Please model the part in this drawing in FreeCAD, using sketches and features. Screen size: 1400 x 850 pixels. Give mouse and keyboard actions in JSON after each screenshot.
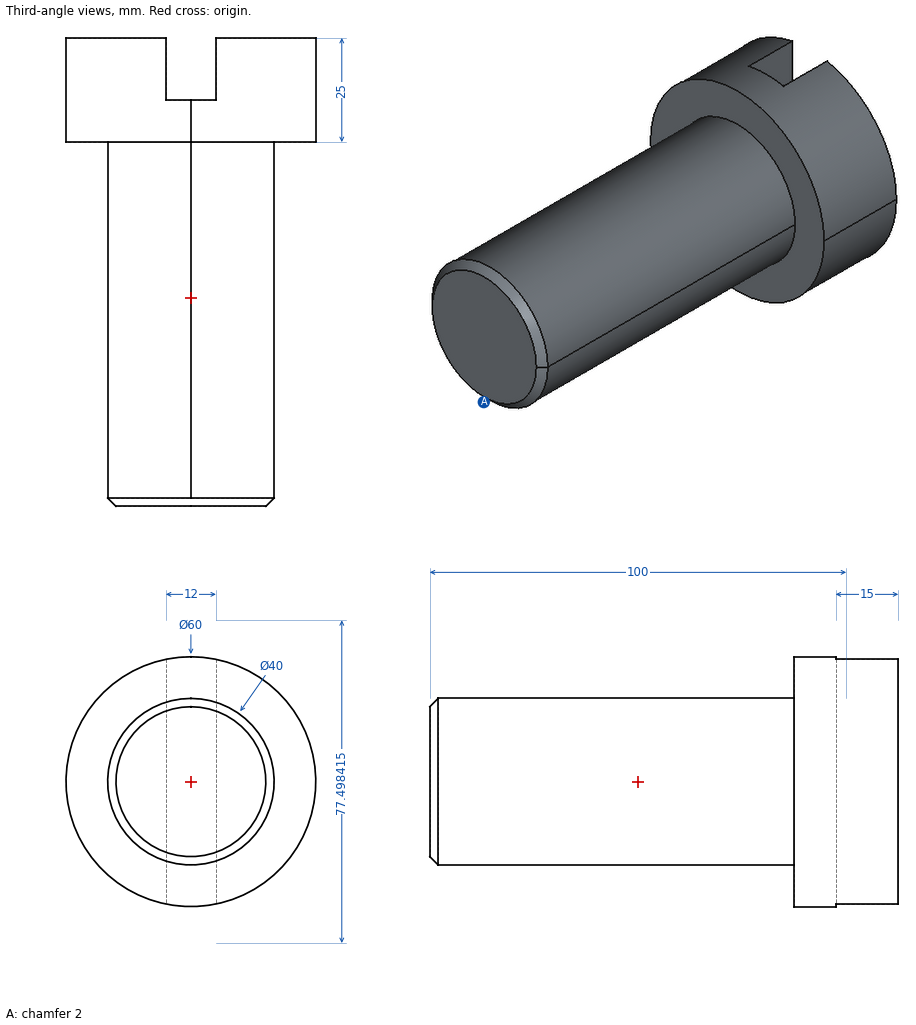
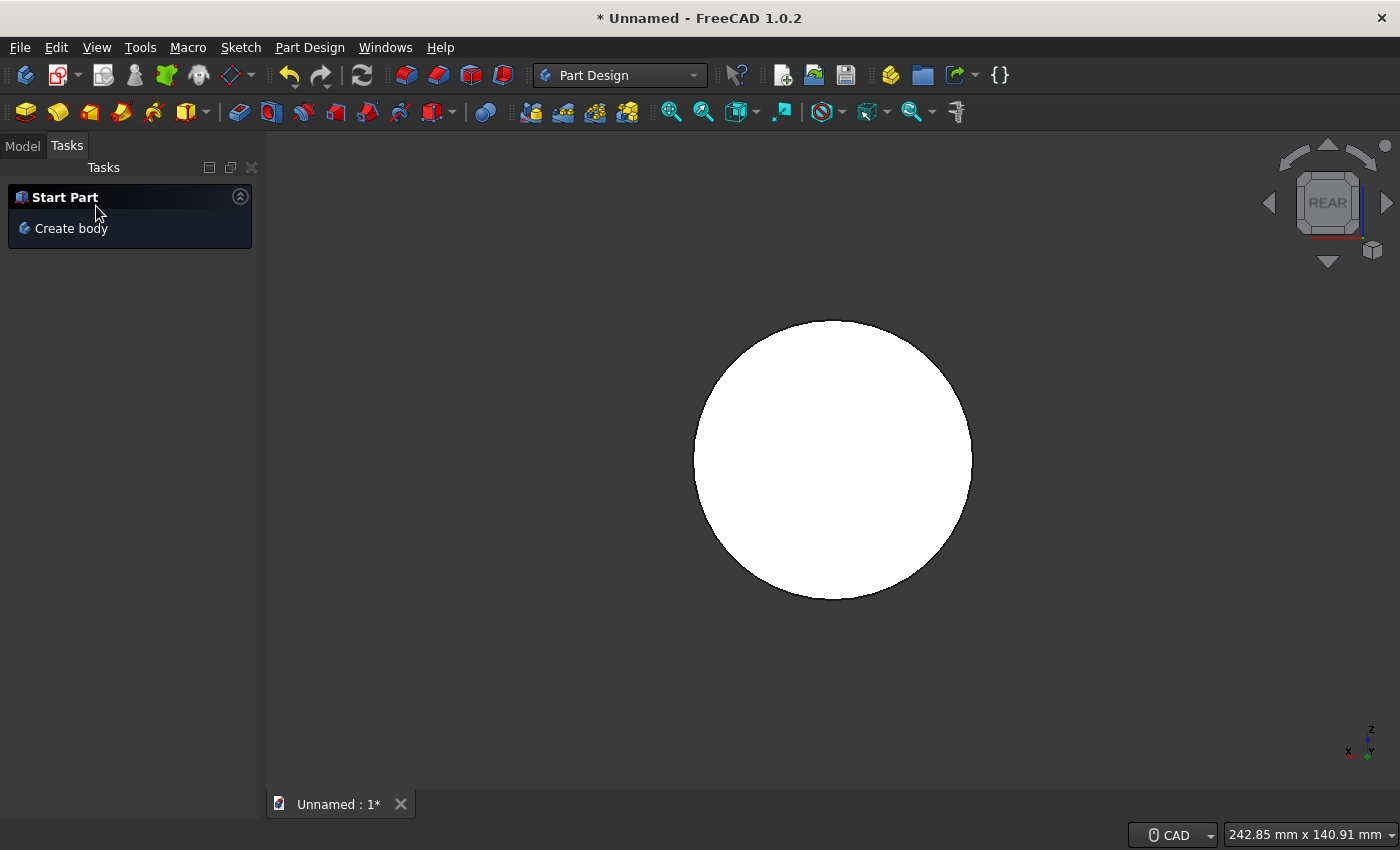
{"action": "left_click", "coordinate": [672, 112]}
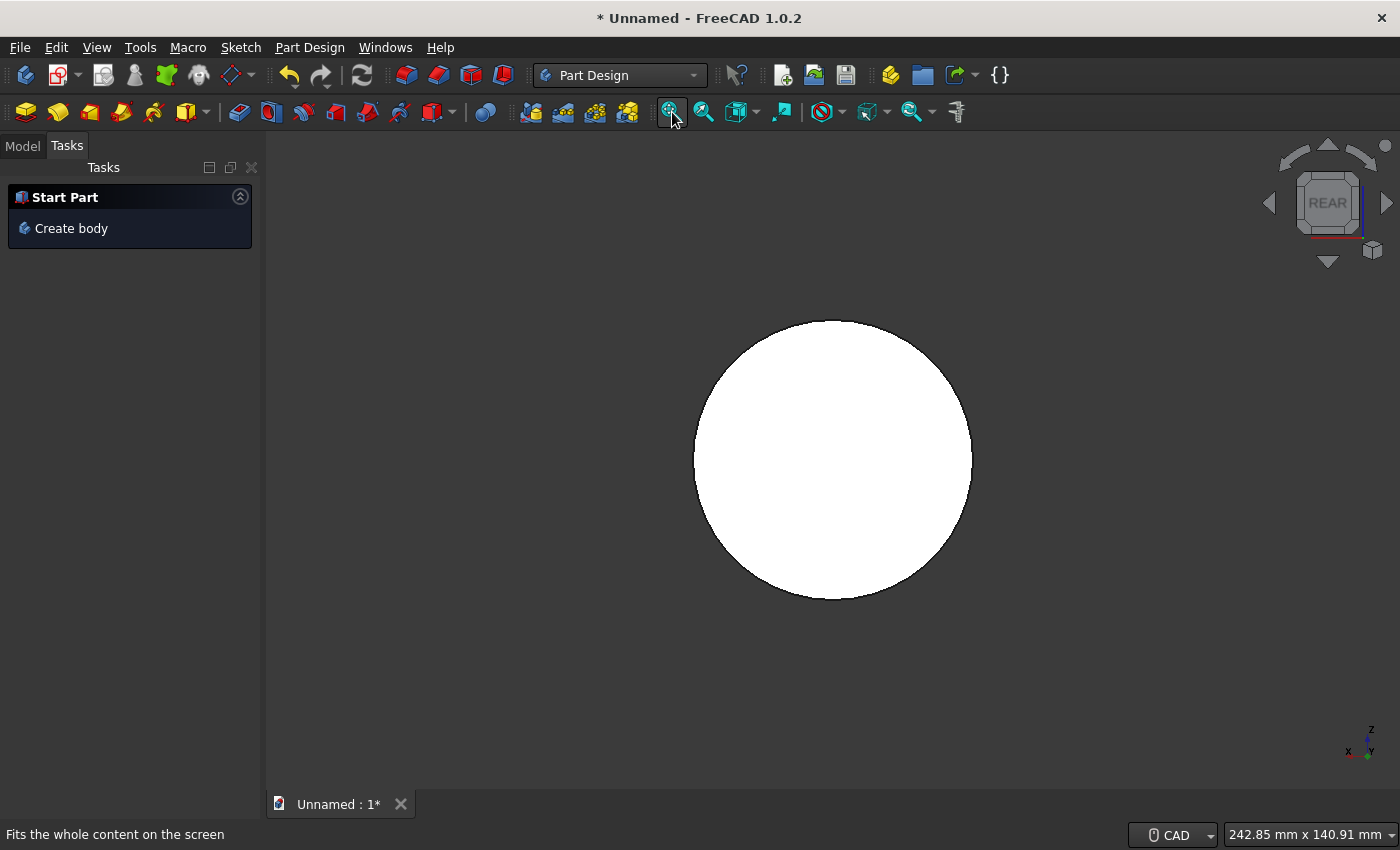
{"action": "left_click", "coordinate": [833, 459]}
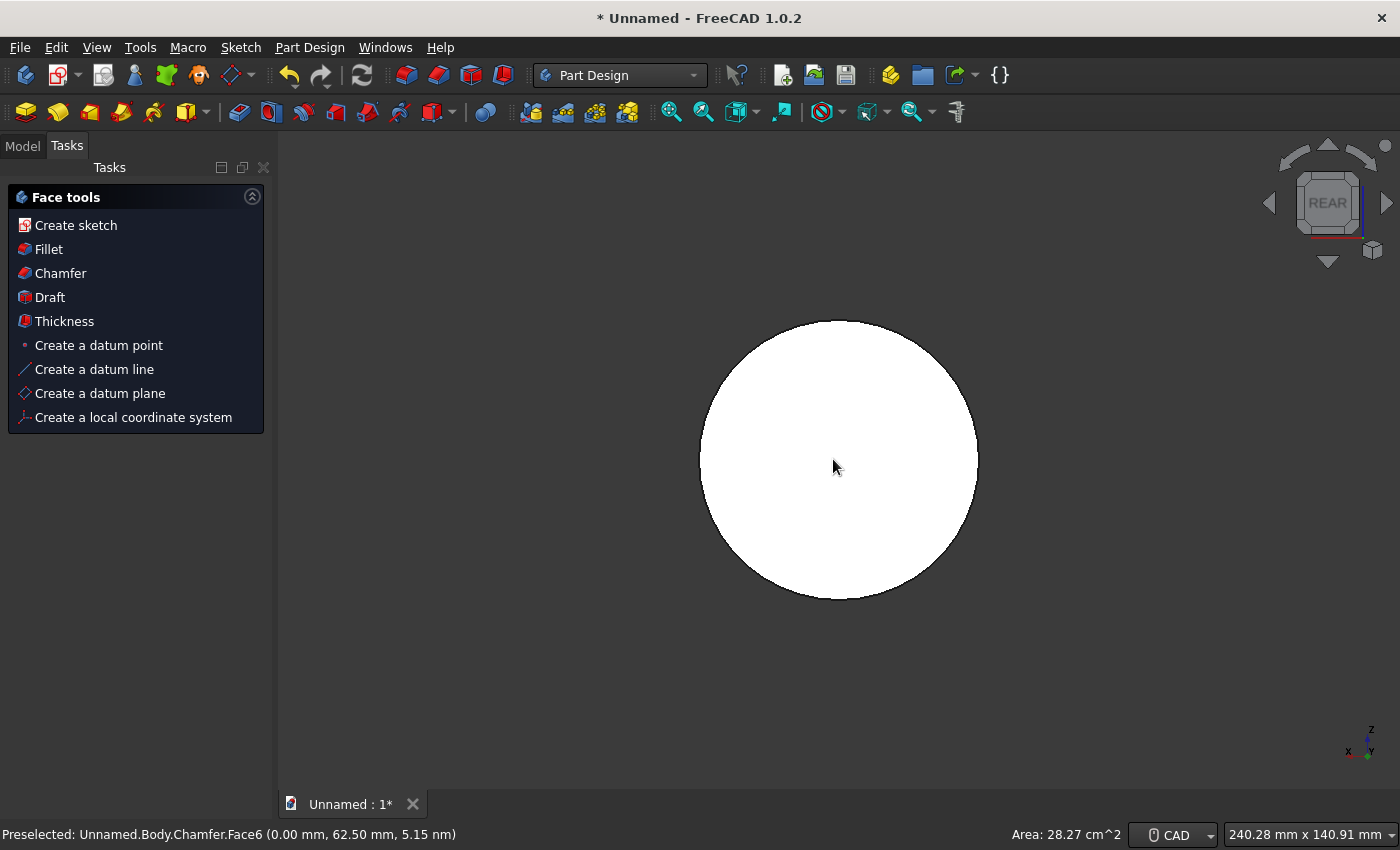
{"action": "left_click", "coordinate": [58, 76]}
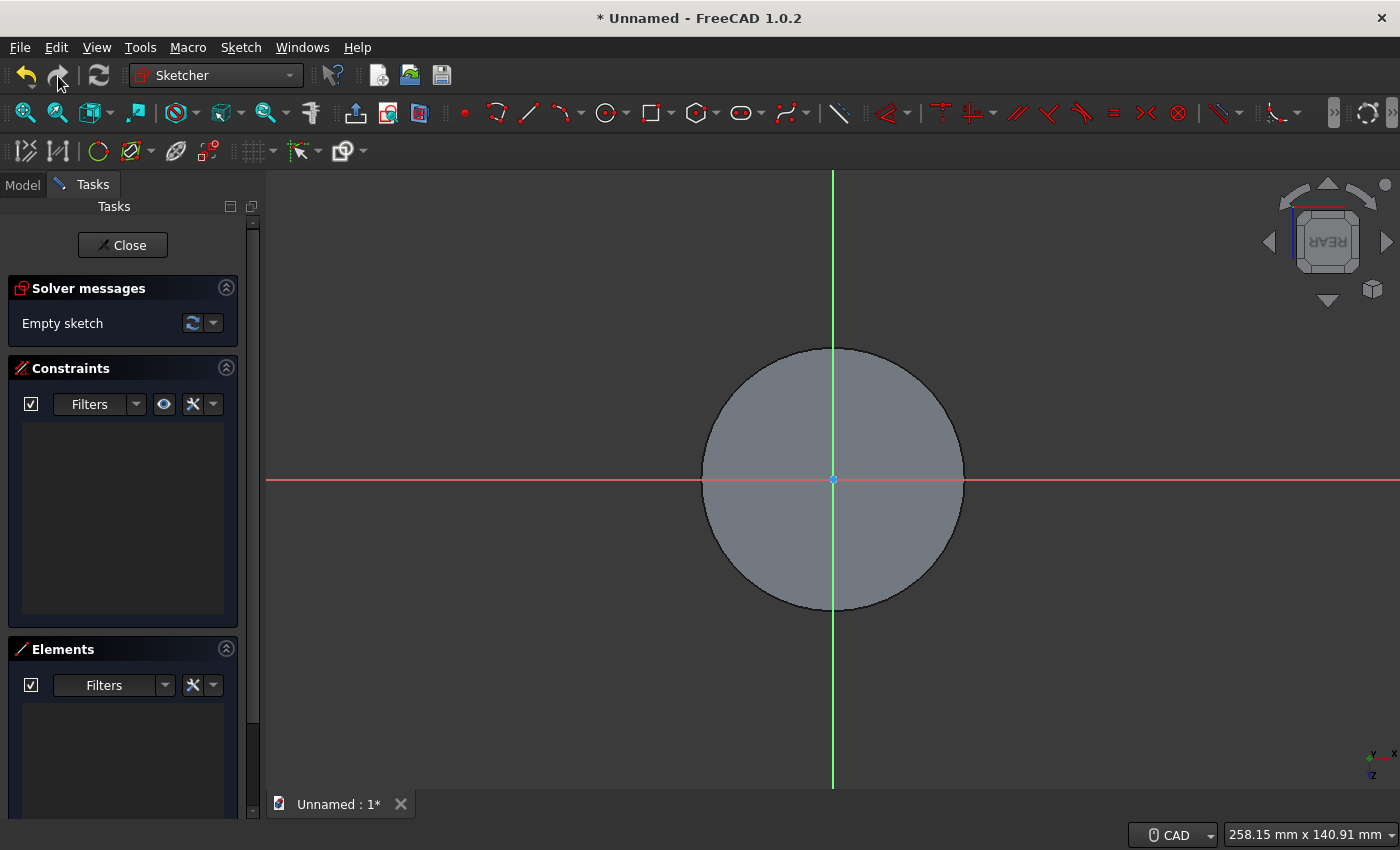
{"action": "left_click", "coordinate": [674, 114]}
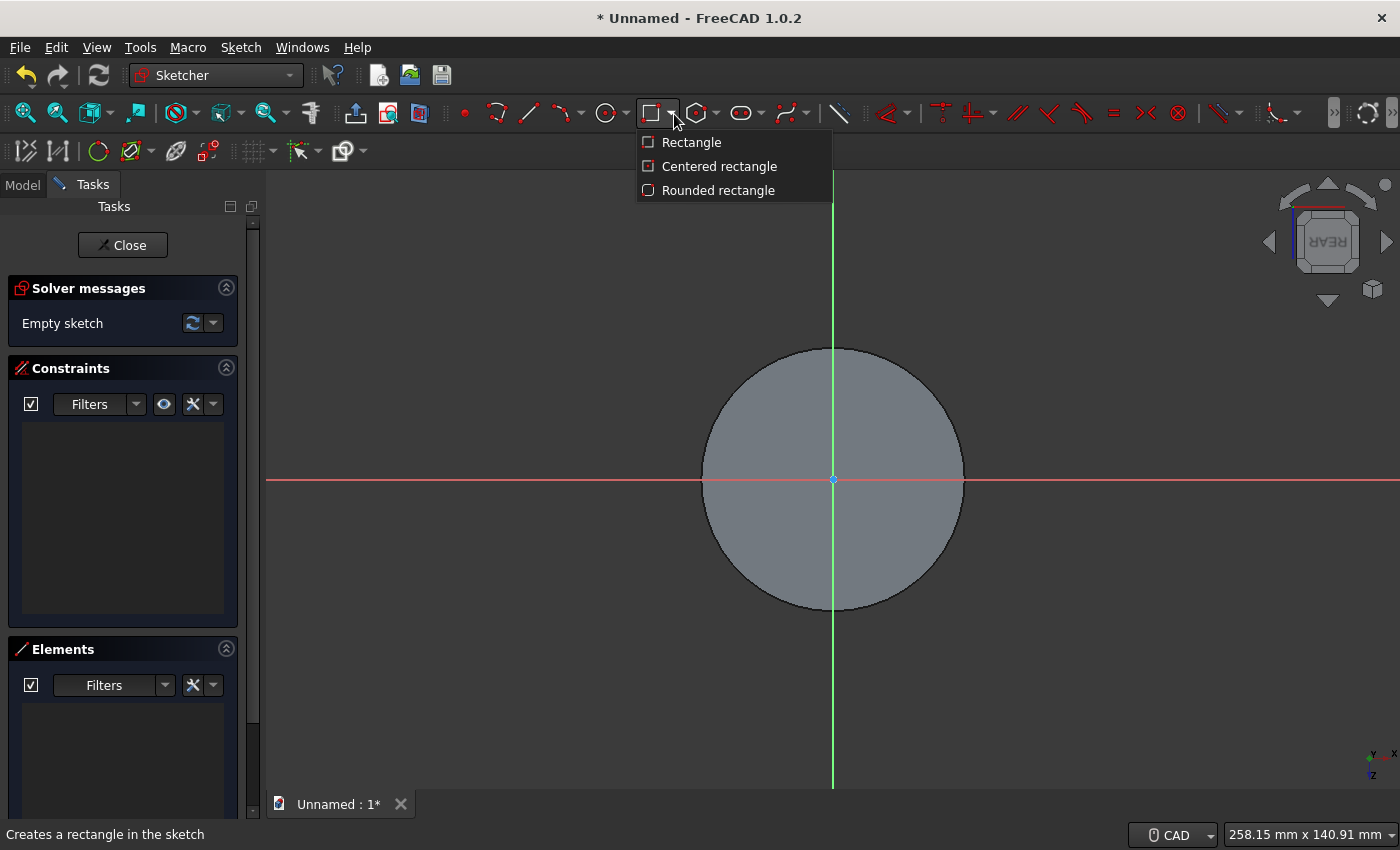
{"action": "left_click", "coordinate": [734, 166]}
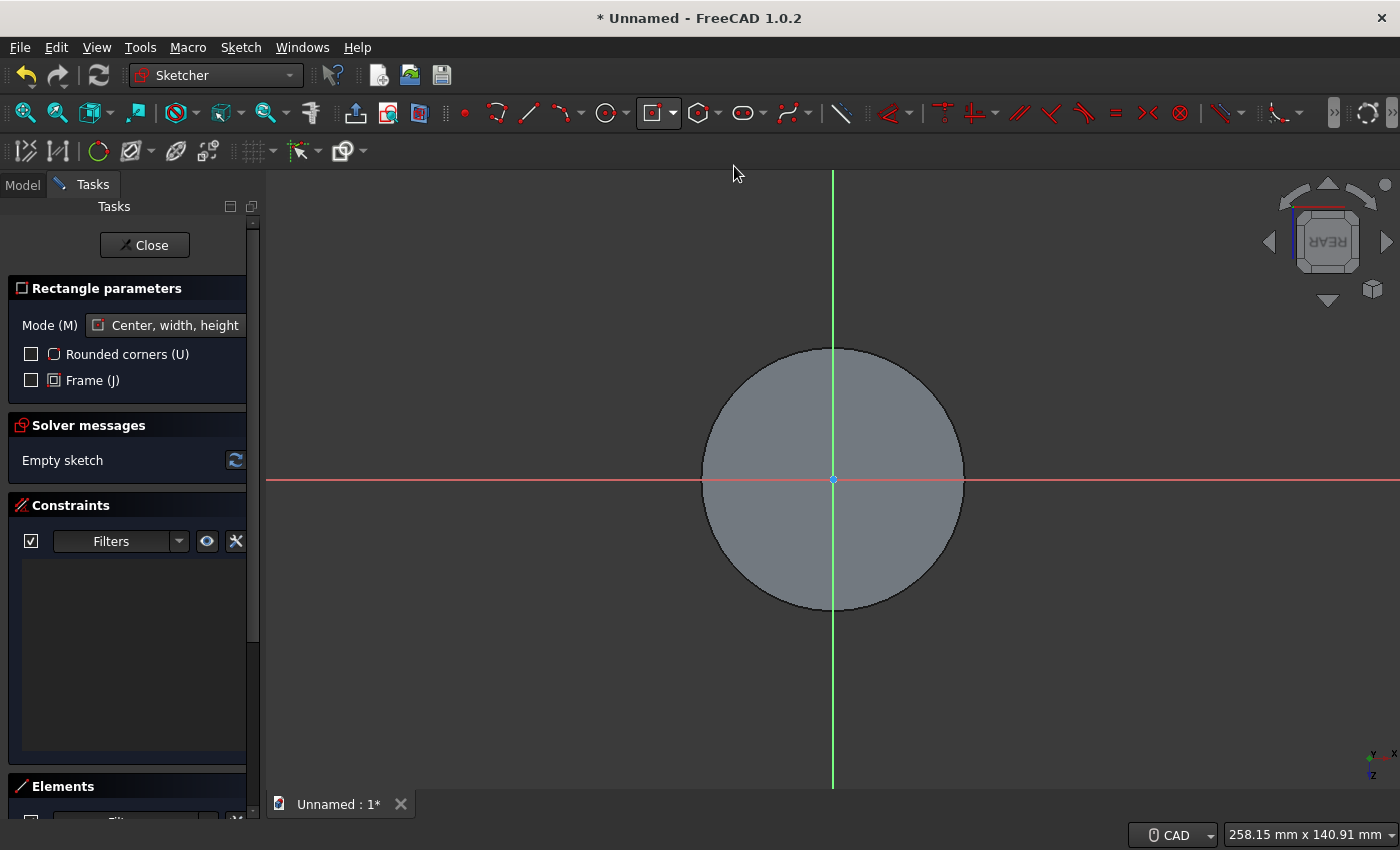
{"action": "left_click", "coordinate": [833, 479]}
{"action": "mouse_move", "coordinate": [859, 309]}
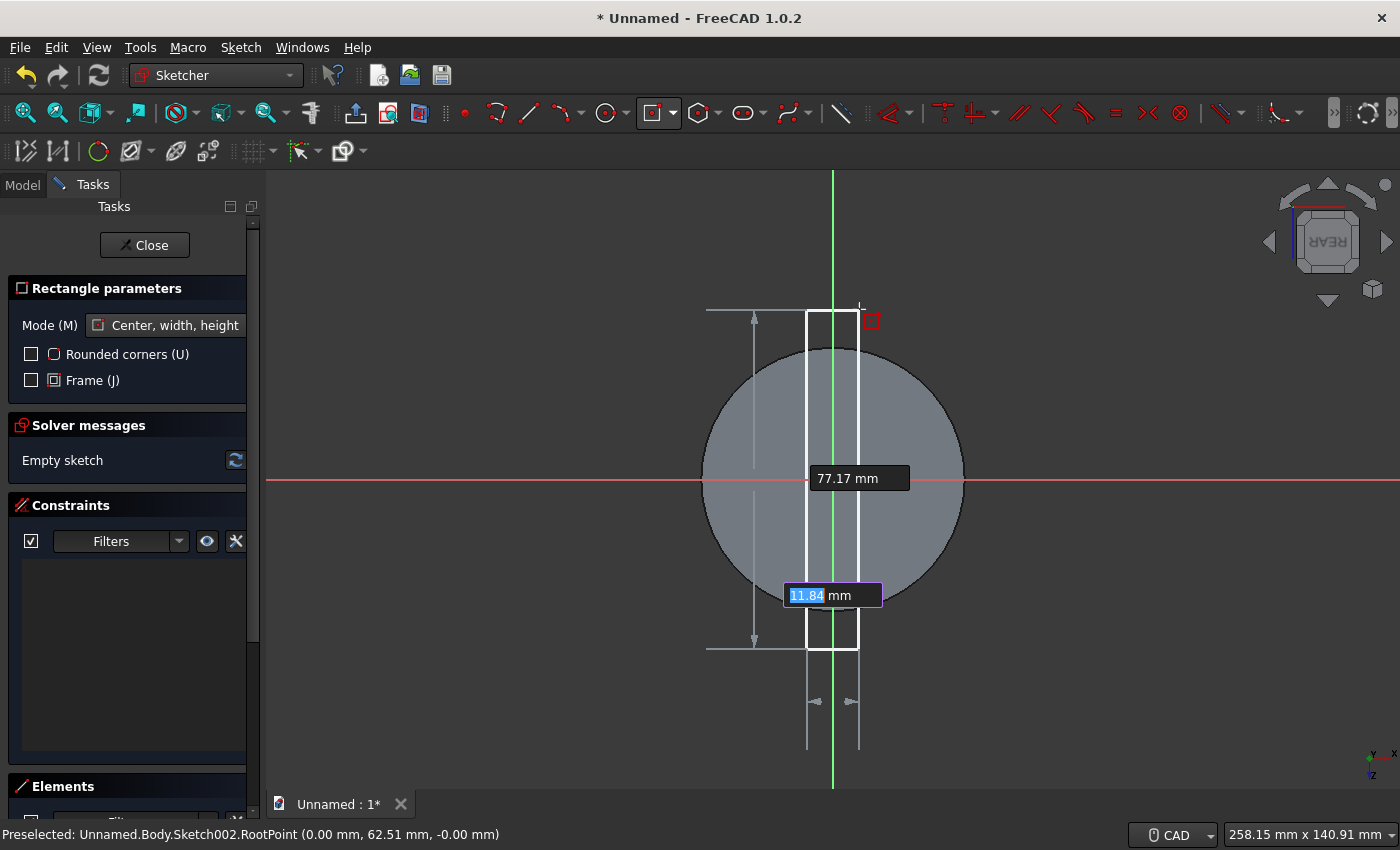
{"action": "type", "text": "12"}
{"action": "key", "text": "Tab"}
{"action": "type", "text": "77.498415"}
{"action": "key", "text": "Return"}
{"action": "key", "text": "Escape"}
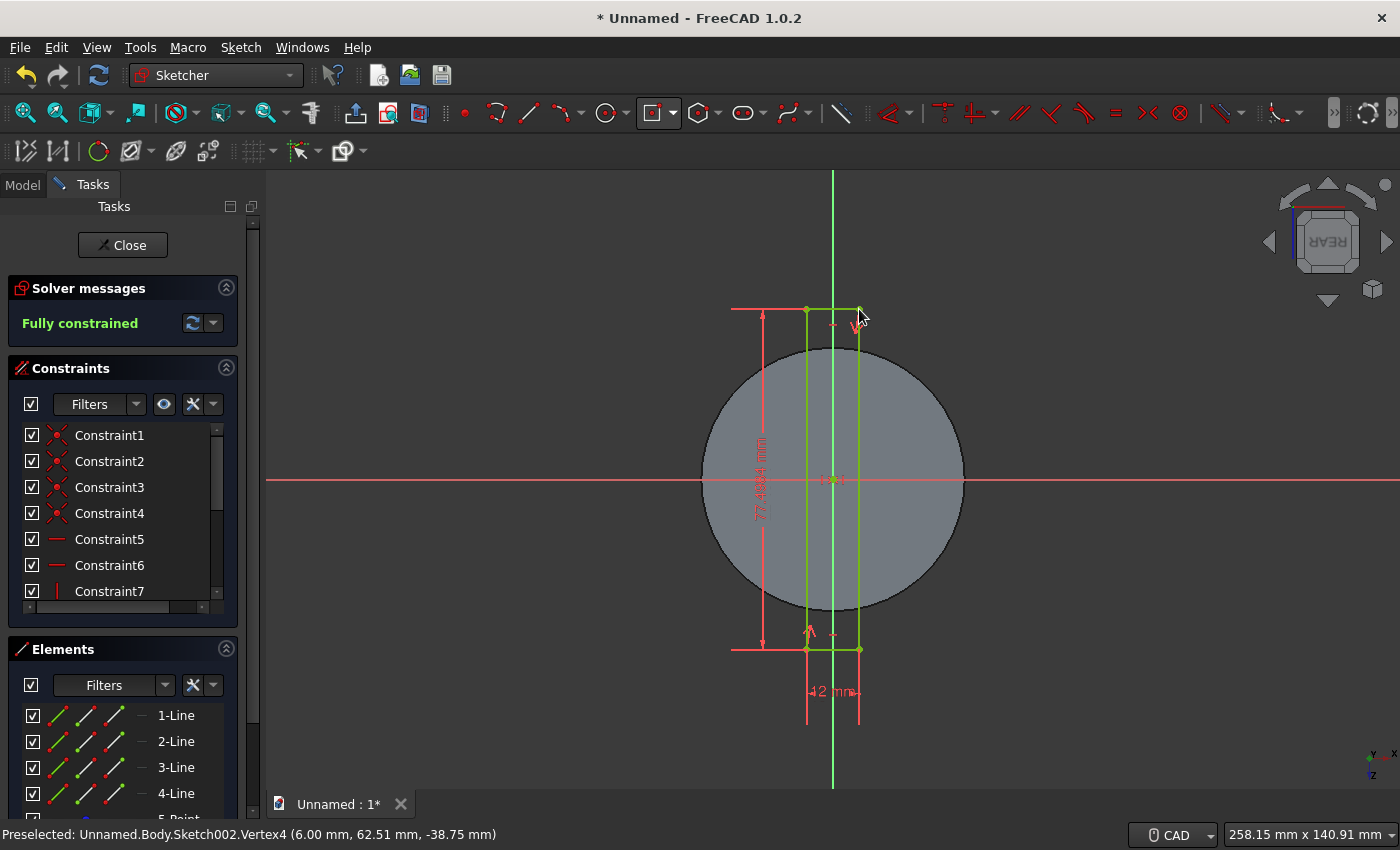
{"action": "left_click", "coordinate": [123, 245]}